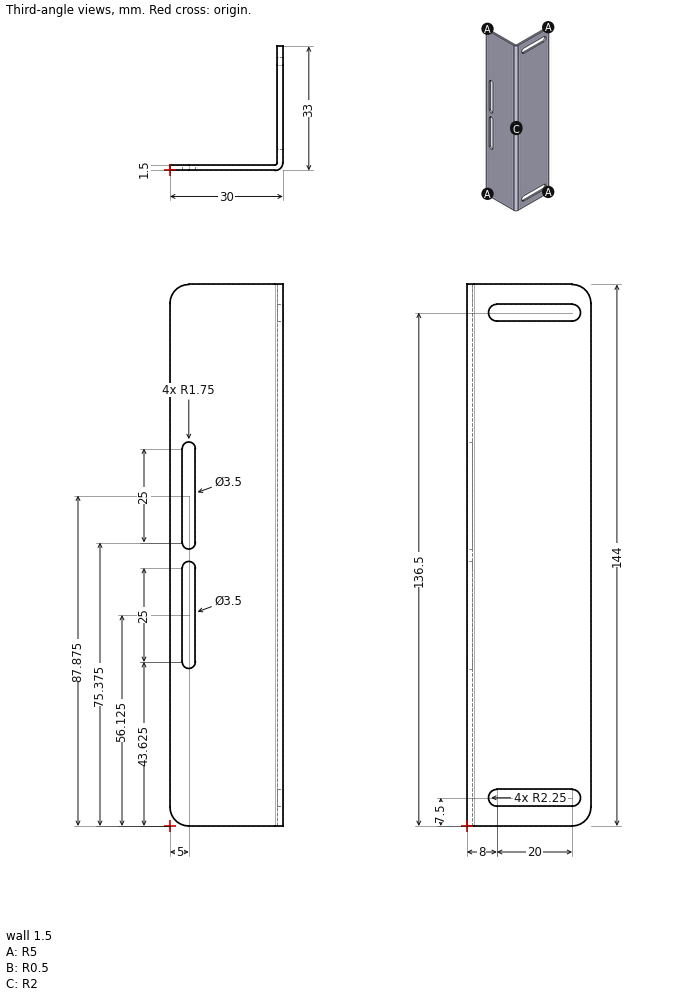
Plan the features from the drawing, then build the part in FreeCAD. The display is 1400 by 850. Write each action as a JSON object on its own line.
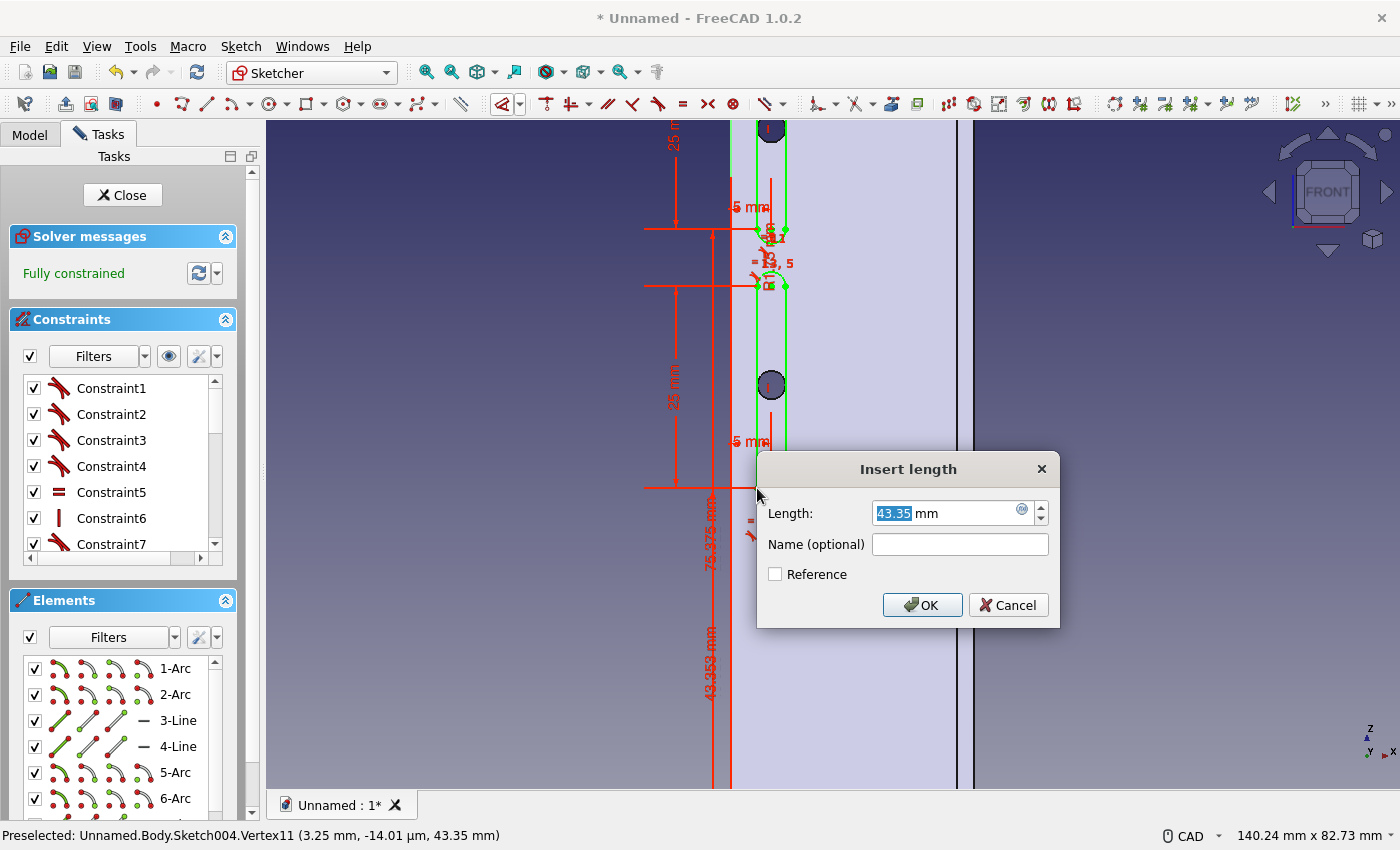
{"action": "type", "text": "43.625"}
{"action": "key", "text": "Return"}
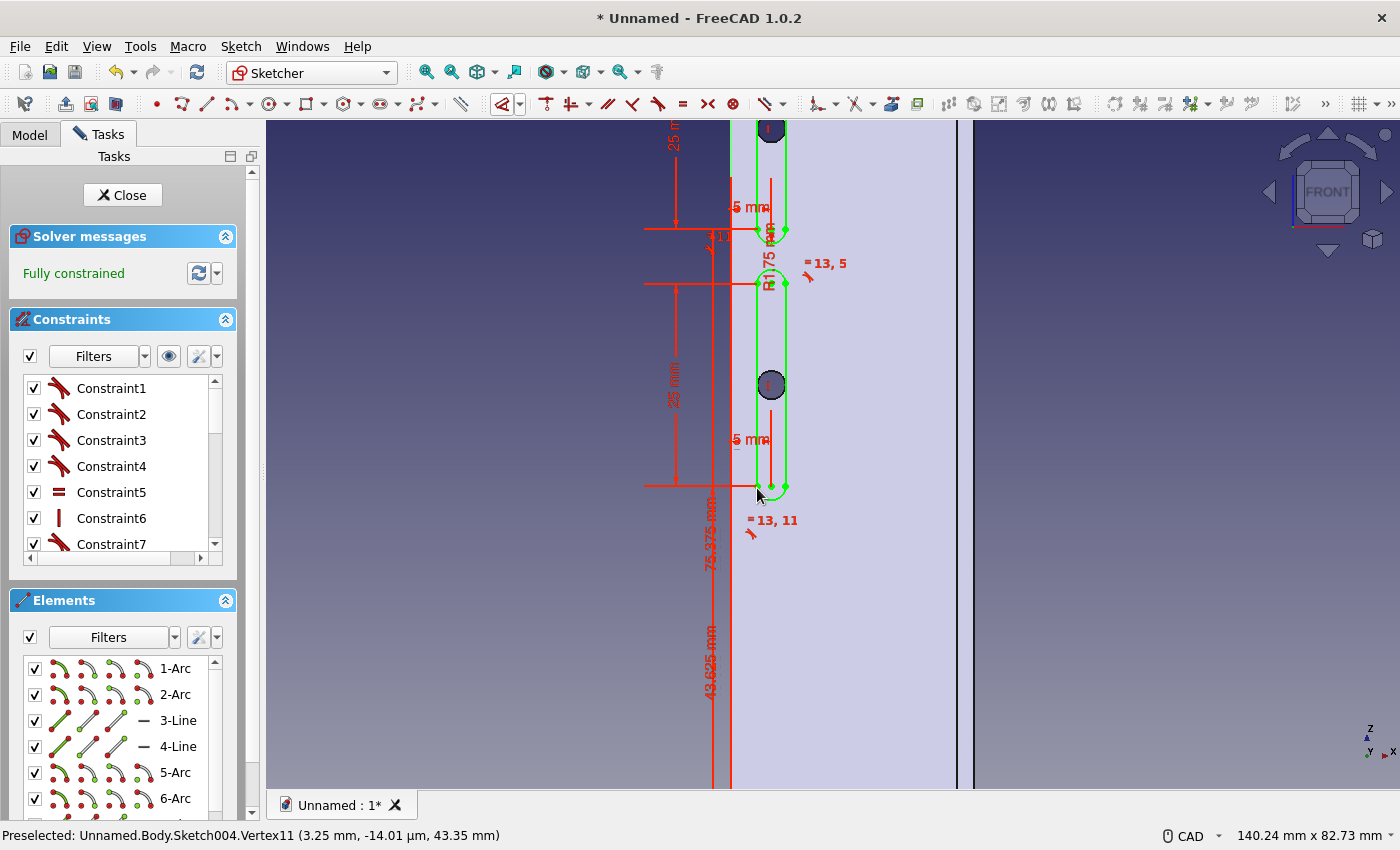
{"action": "left_click", "coordinate": [123, 195]}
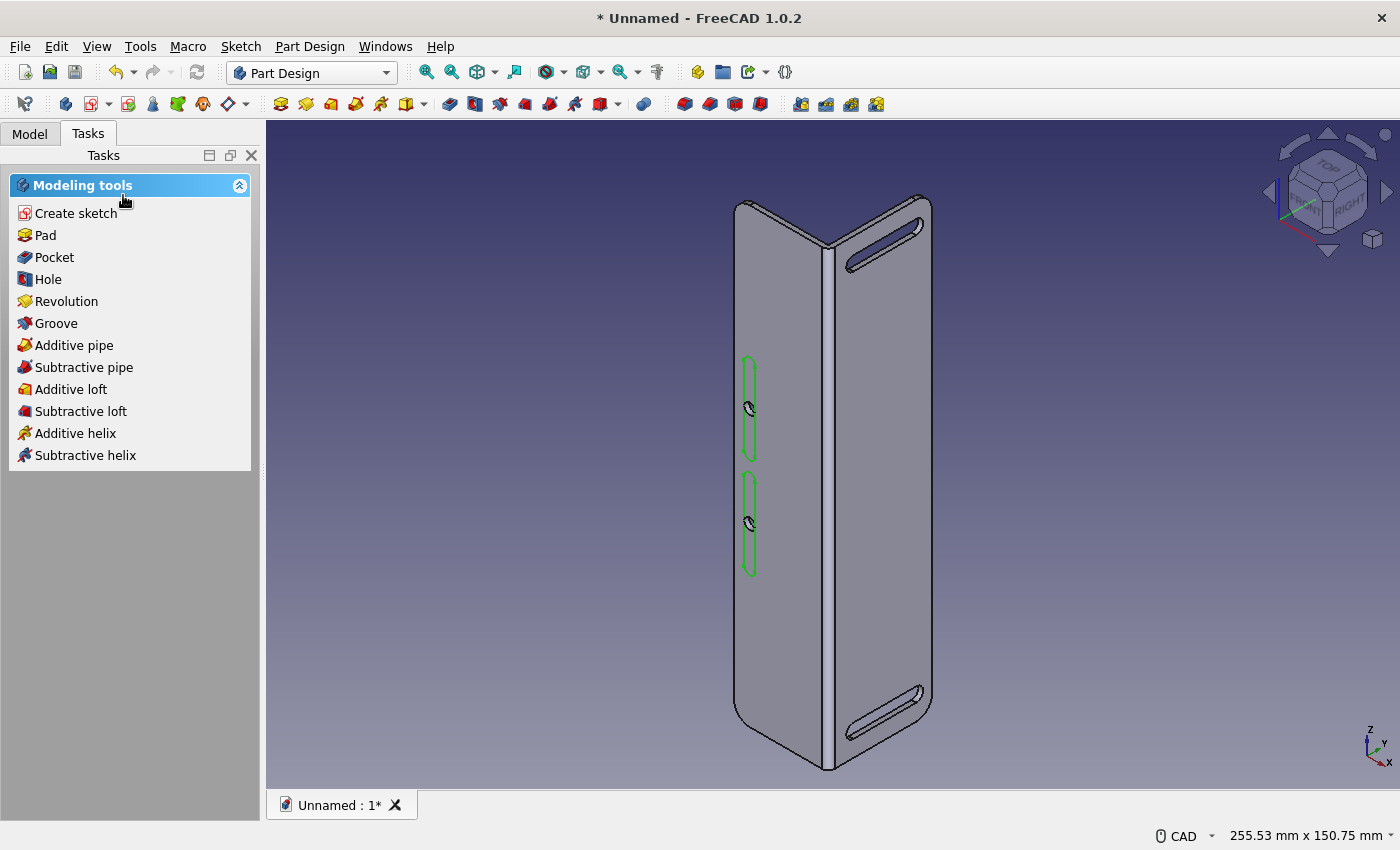
{"action": "left_click", "coordinate": [450, 104]}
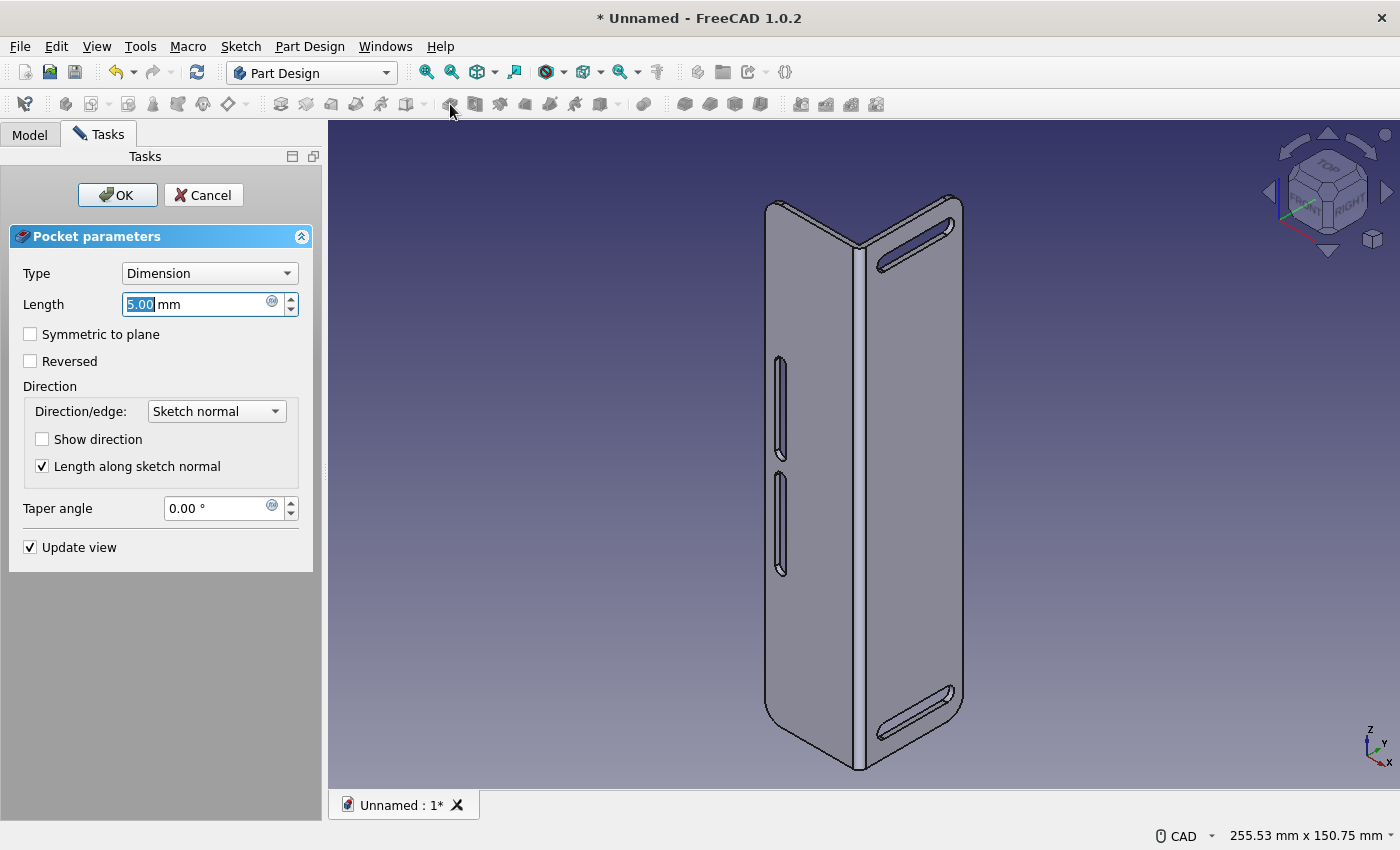
{"action": "type", "text": "1.5"}
{"action": "key", "text": "Tab"}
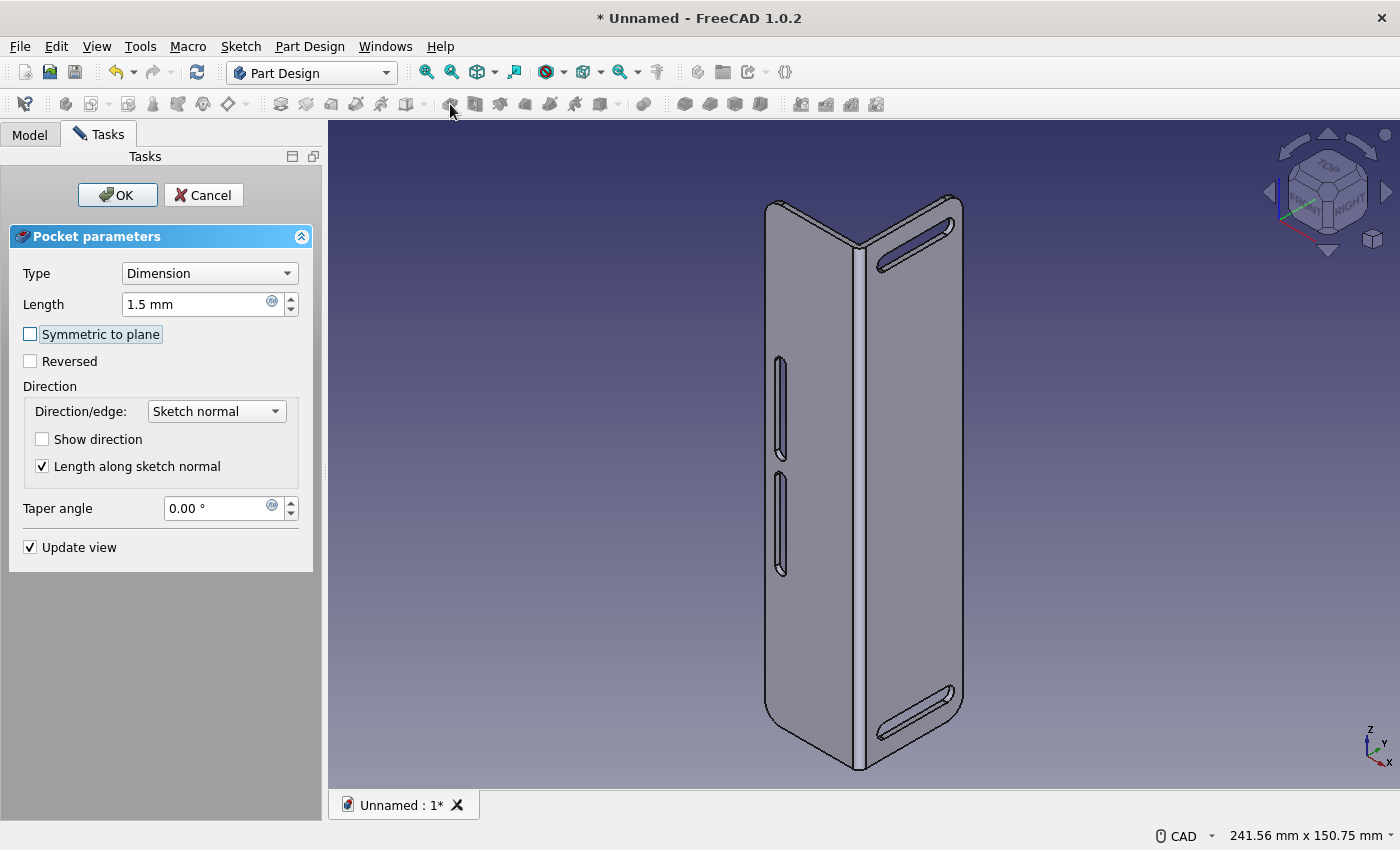
{"action": "left_click", "coordinate": [118, 195]}